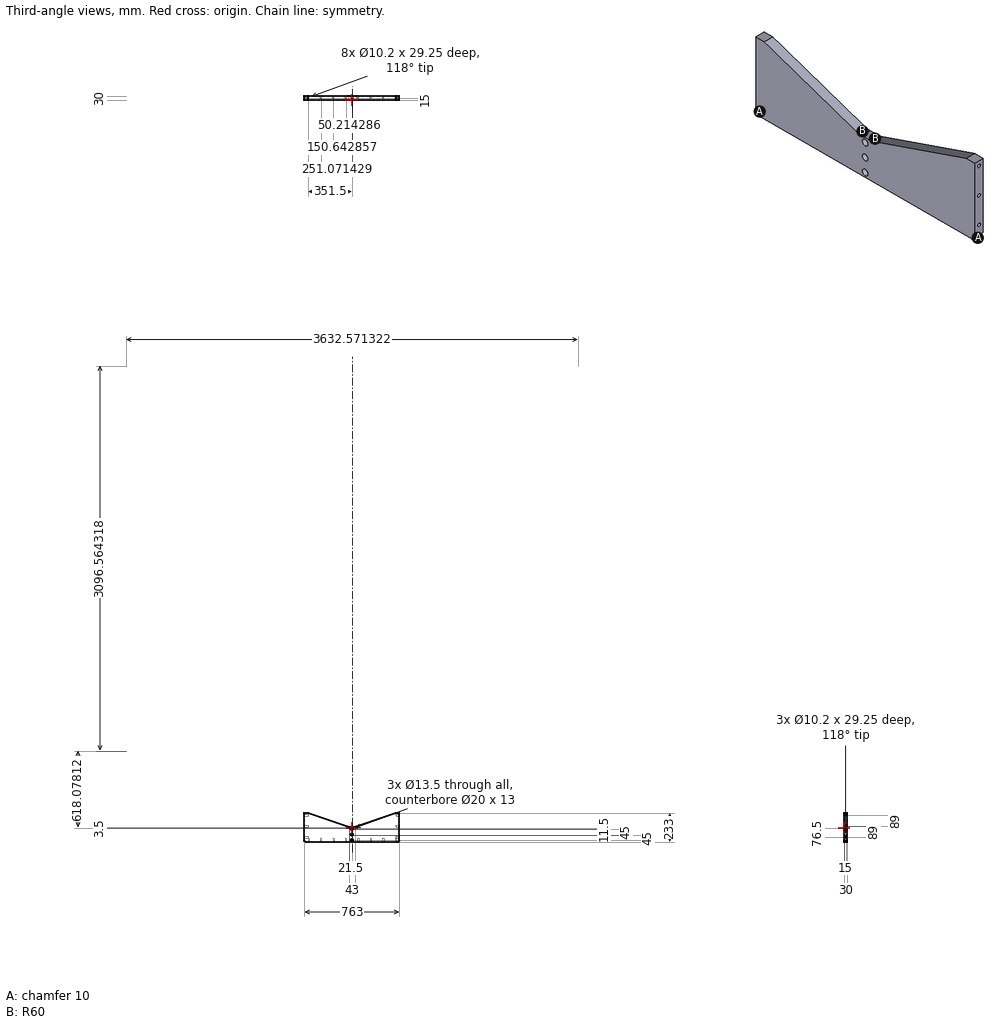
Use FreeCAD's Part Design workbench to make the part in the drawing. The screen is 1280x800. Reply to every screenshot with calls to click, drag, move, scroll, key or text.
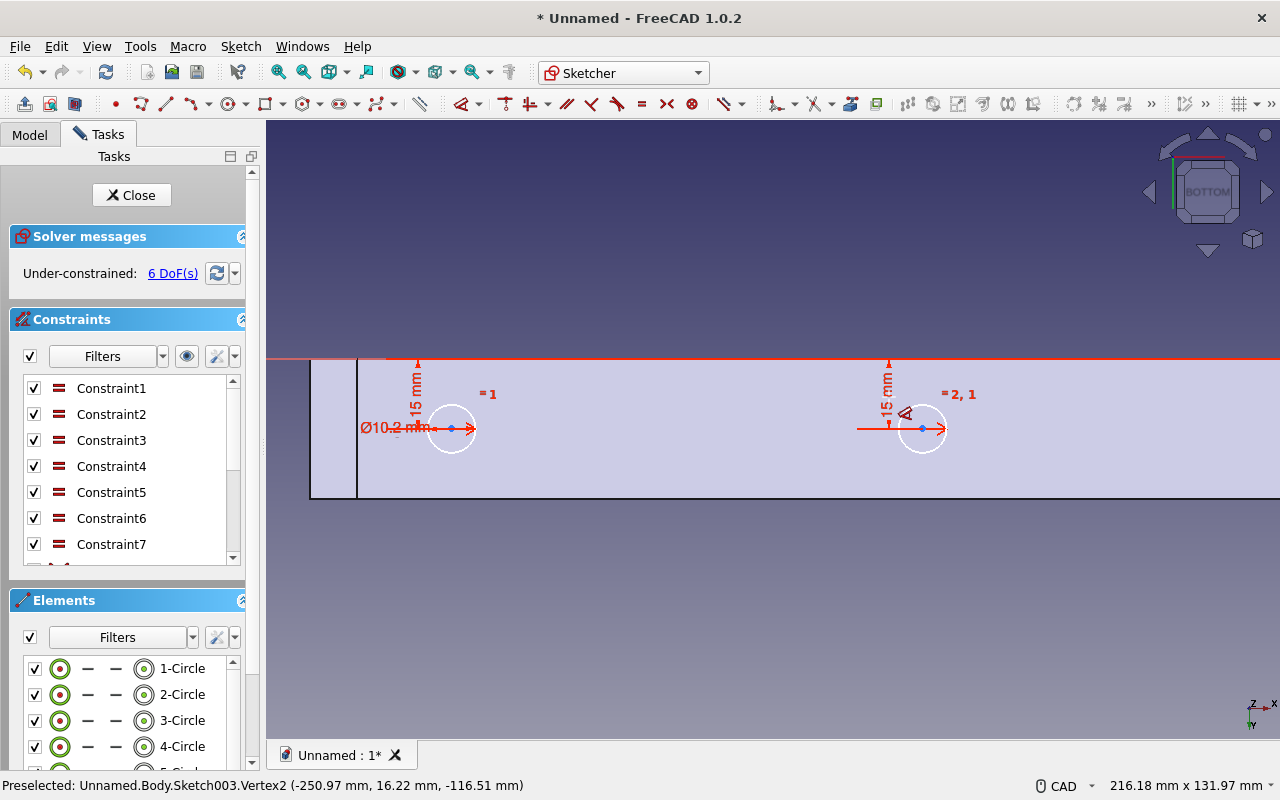
scroll(428, 434, down, 9)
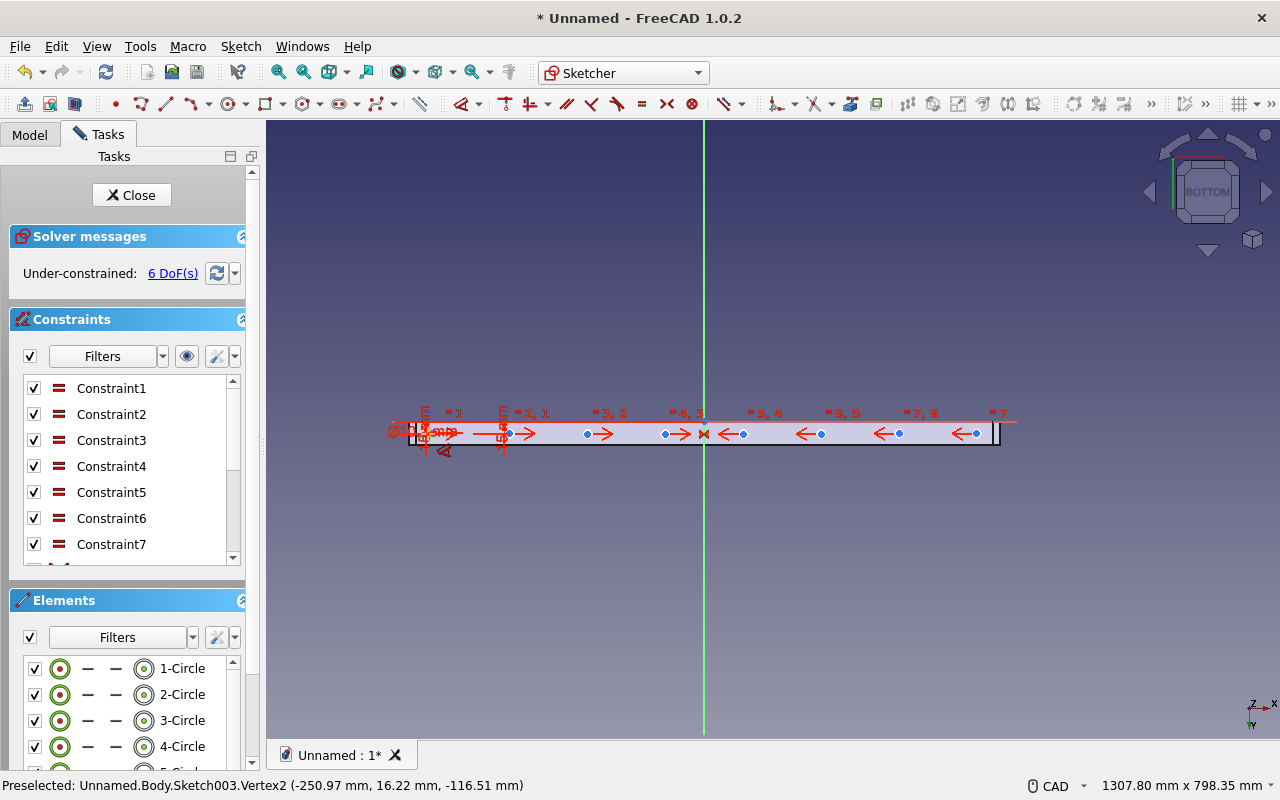
scroll(588, 434, up, 7)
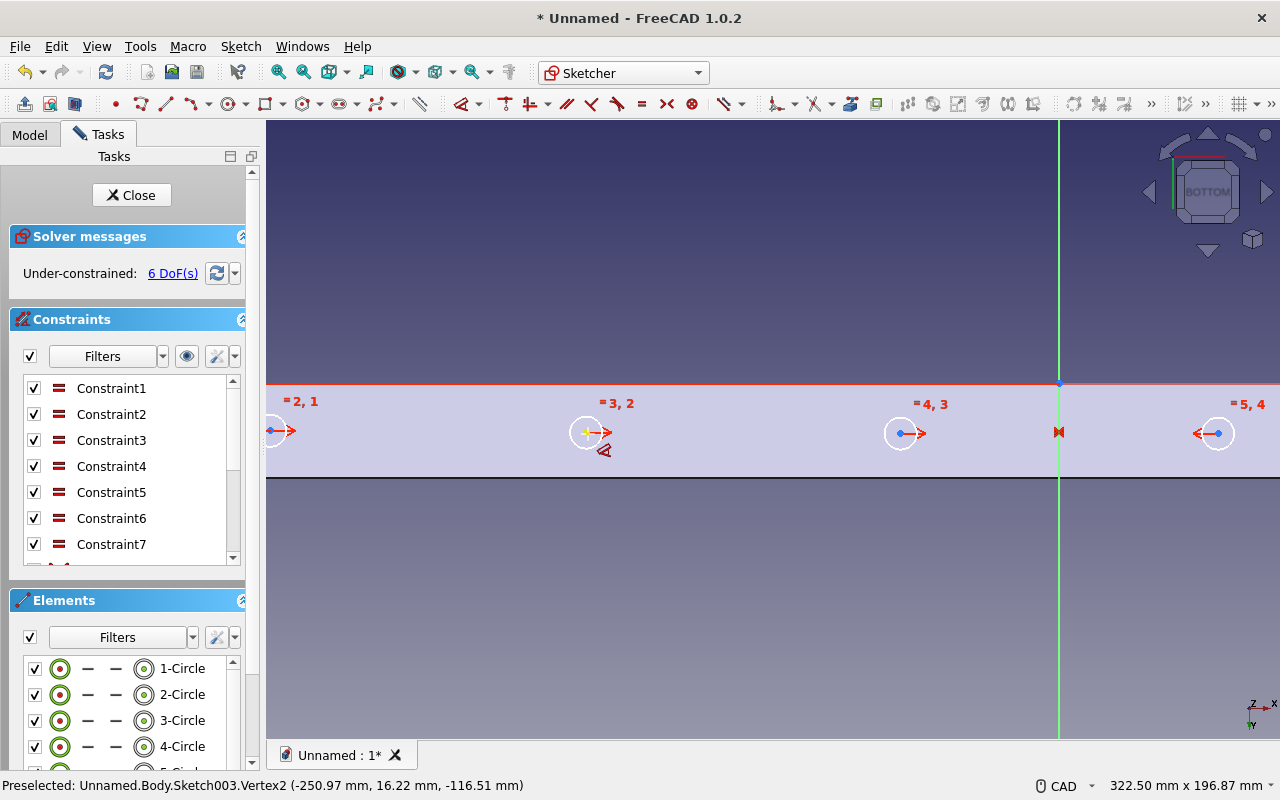
click(586, 433)
click(552, 408)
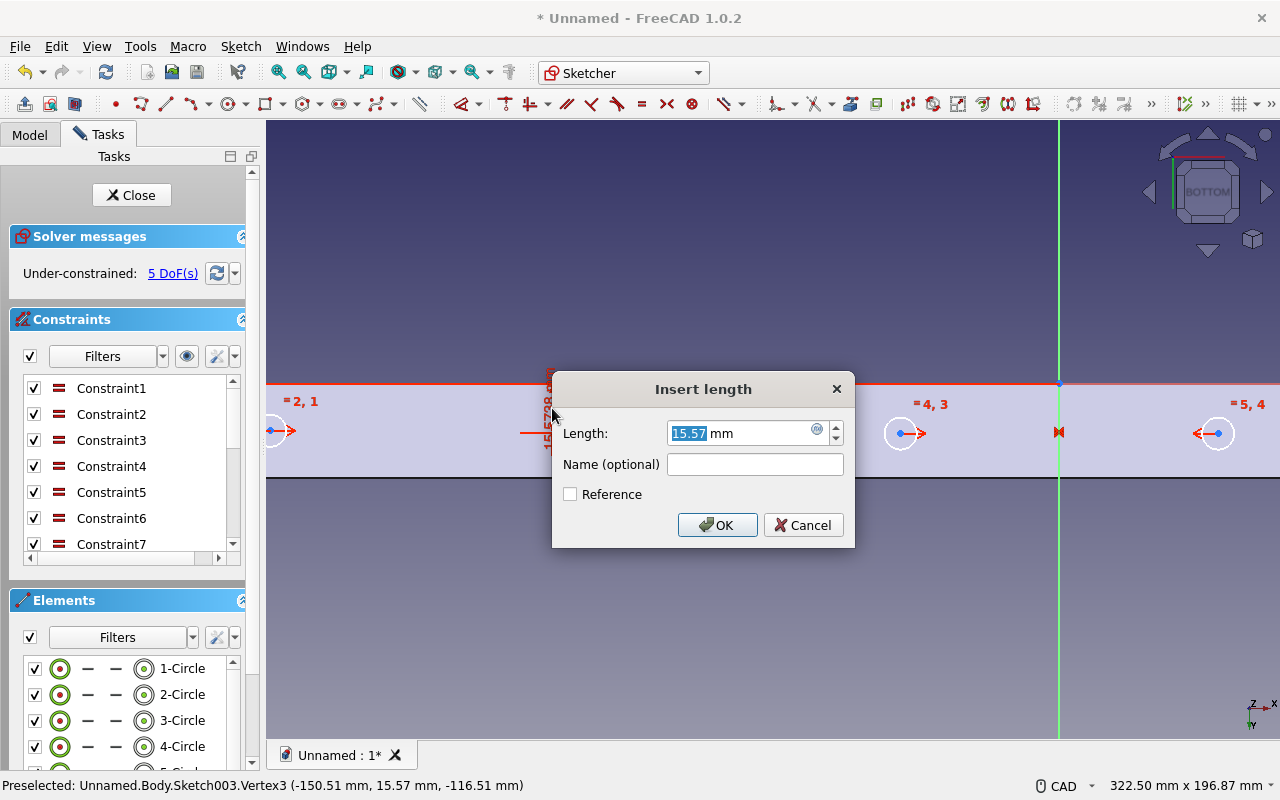
text(15)
key(Return)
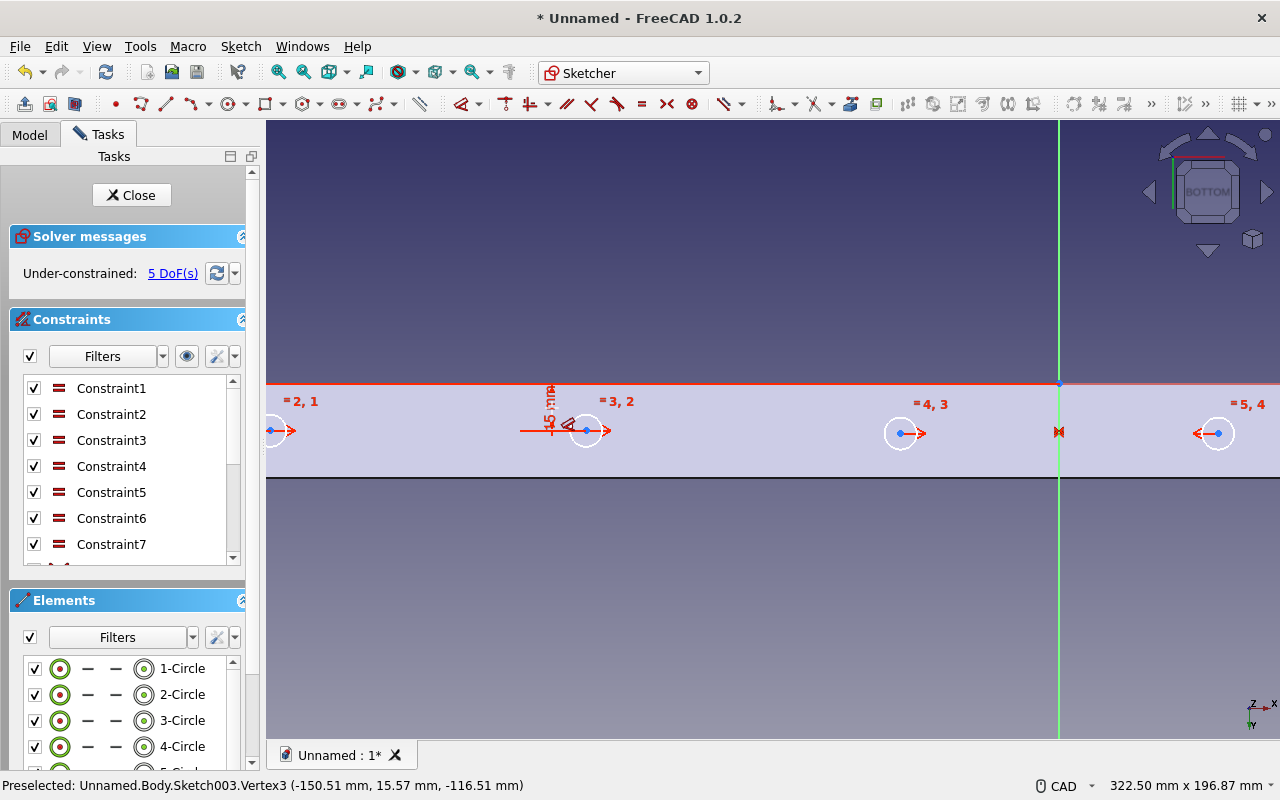
click(901, 434)
click(867, 409)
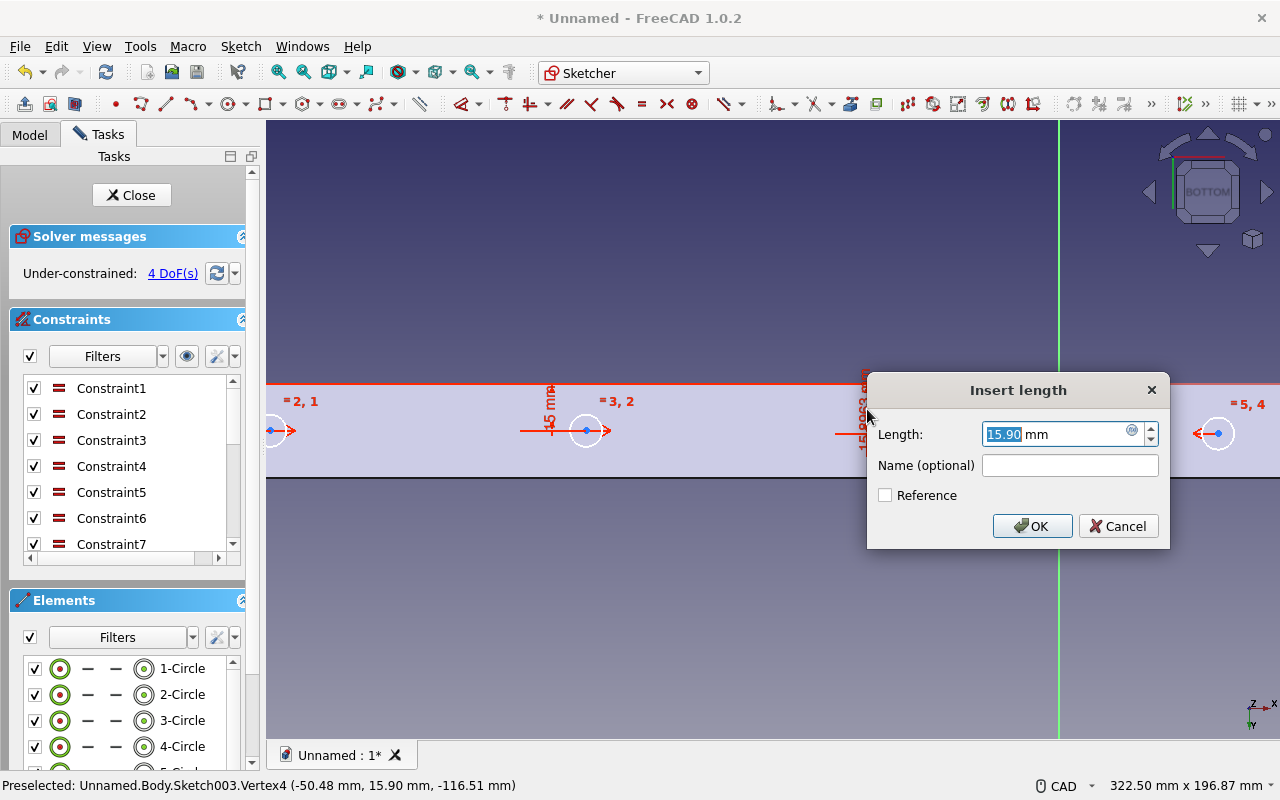
text(15)
key(Return)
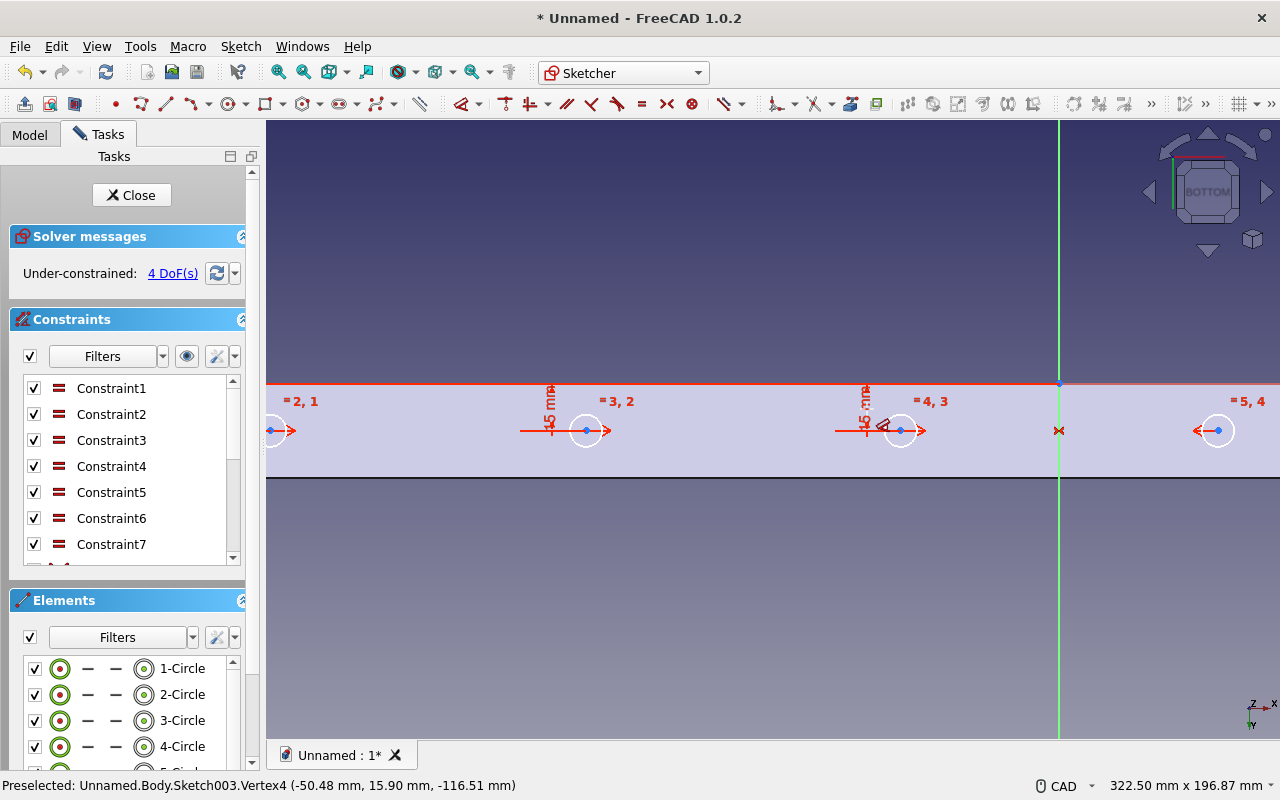
scroll(588, 434, down, 7)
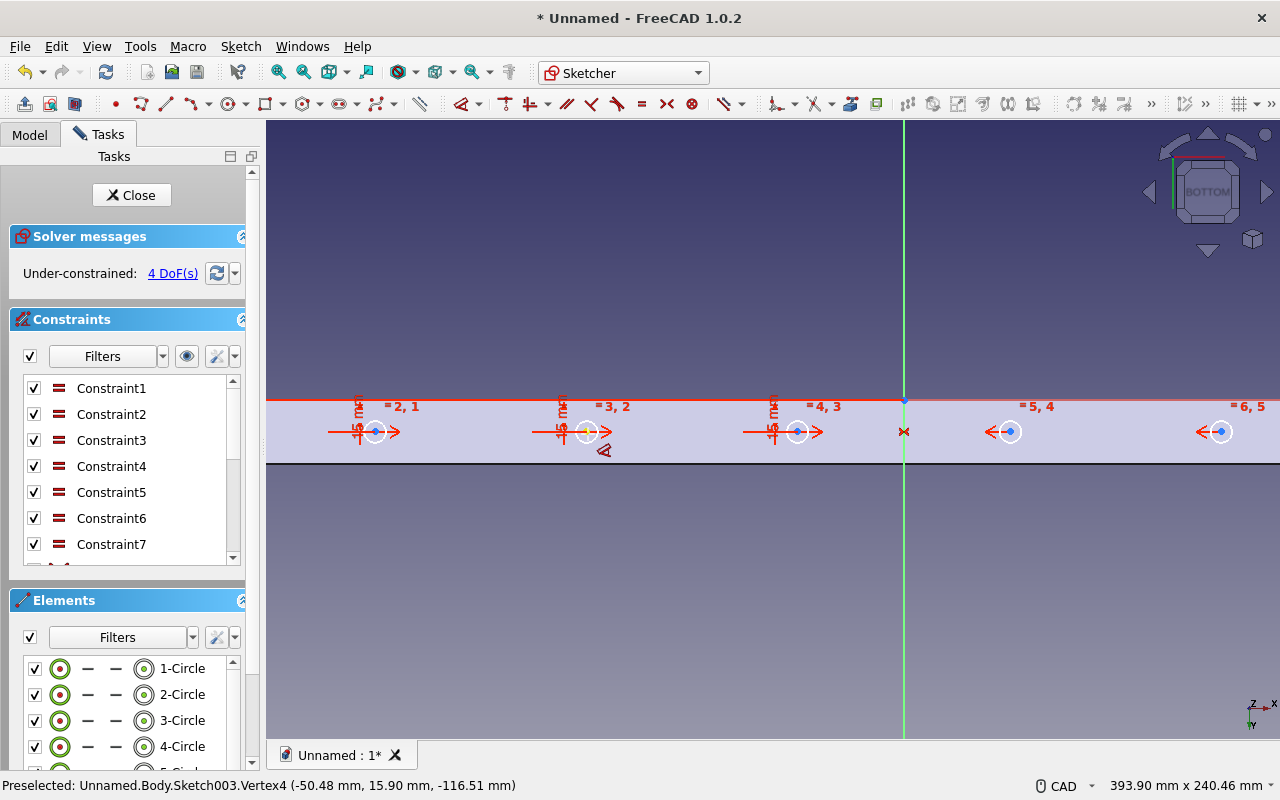
click(432, 434)
click(568, 388)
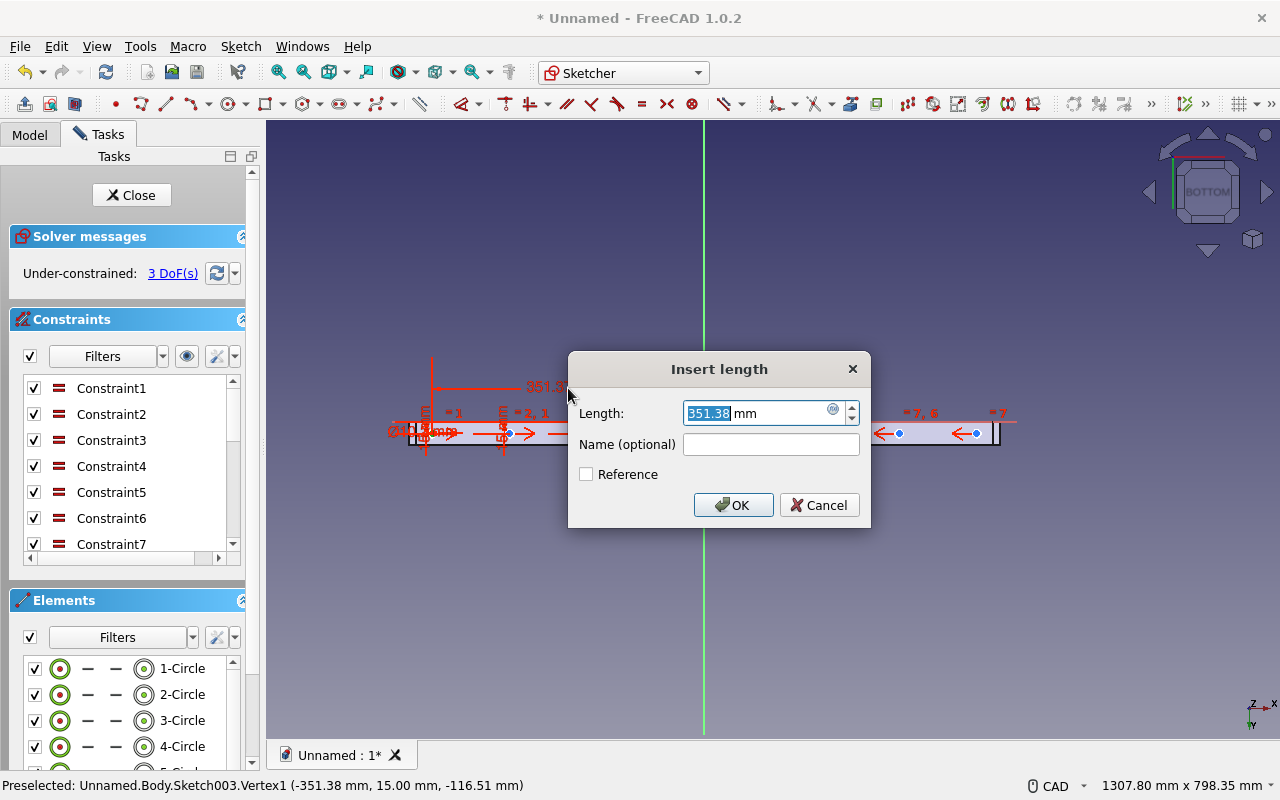
text(351.5)
key(Return)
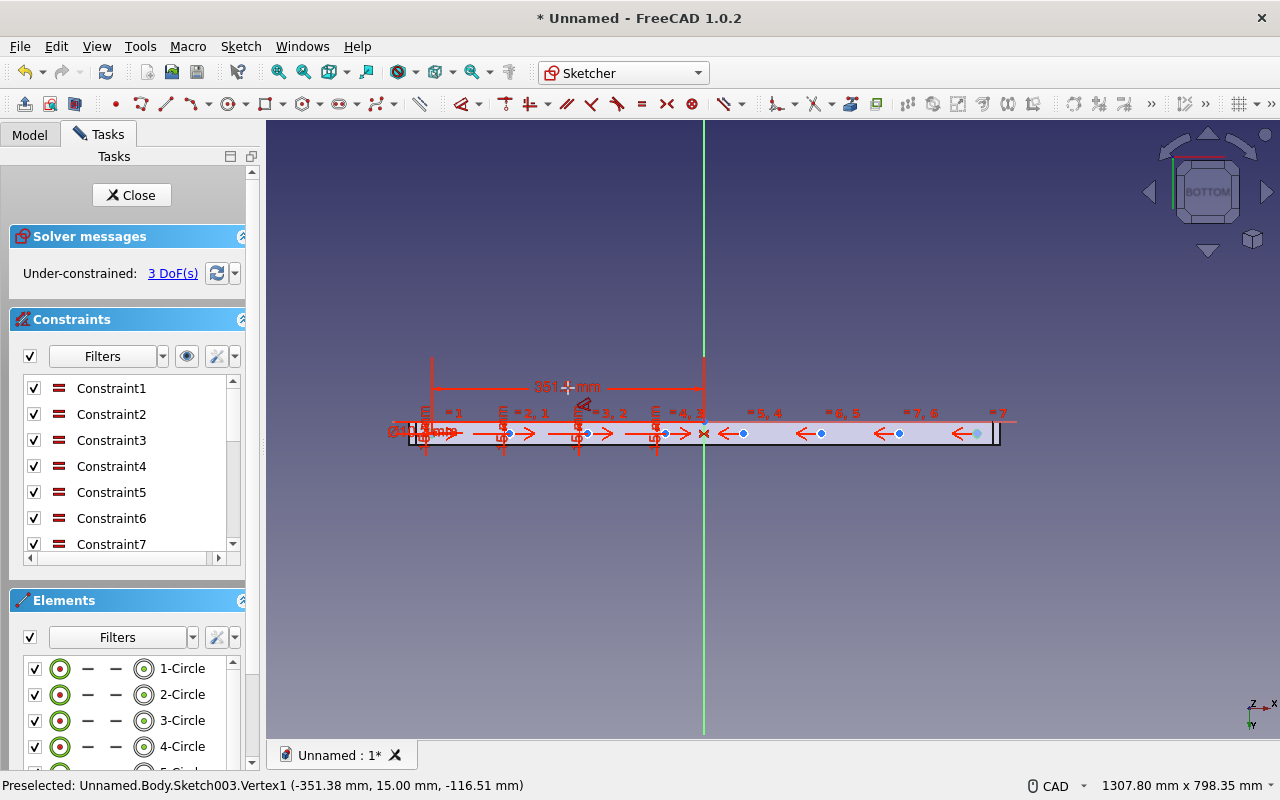
click(665, 434)
click(685, 388)